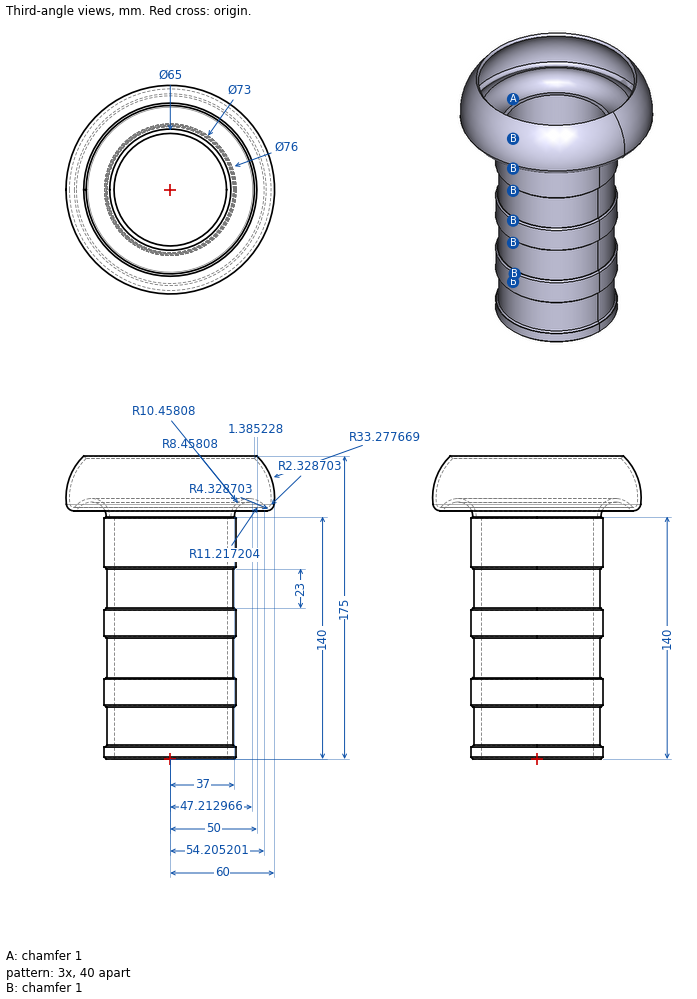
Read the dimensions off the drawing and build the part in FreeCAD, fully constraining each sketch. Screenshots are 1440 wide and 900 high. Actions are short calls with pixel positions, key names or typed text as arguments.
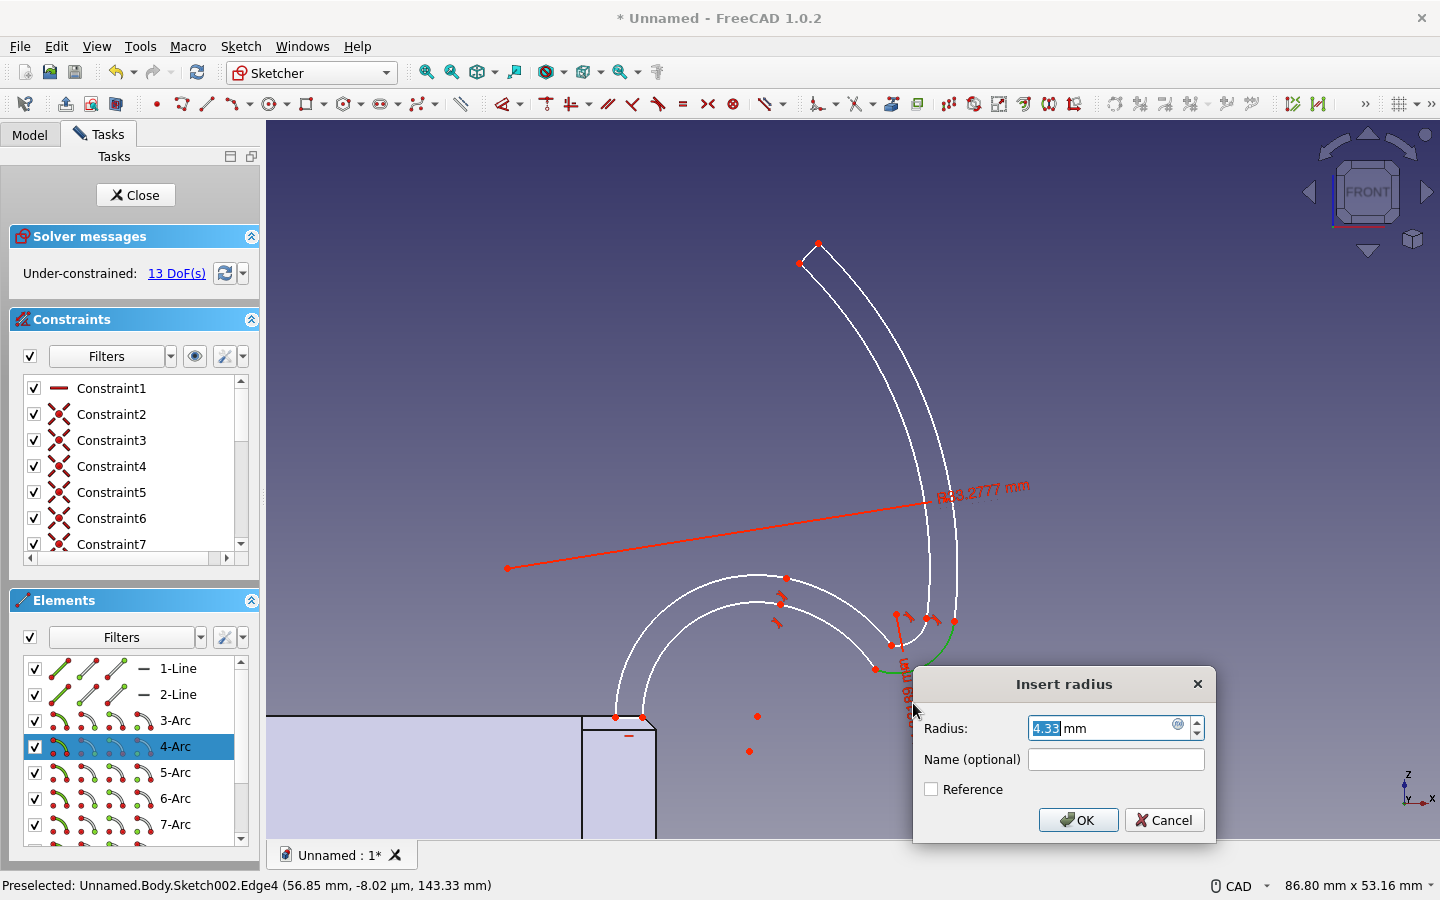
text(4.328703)
key(Return)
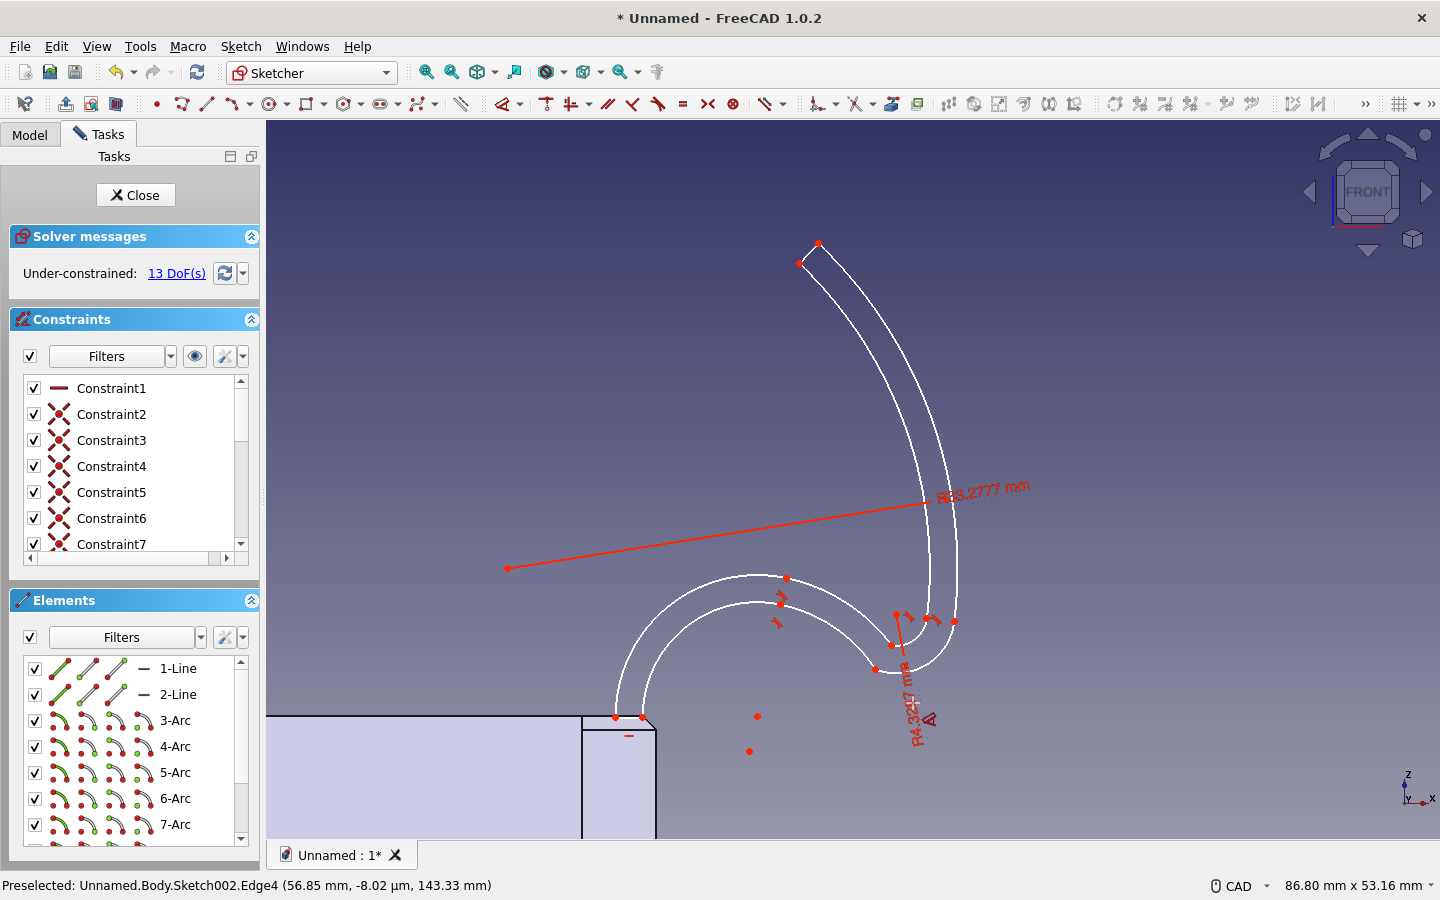
click(853, 643)
click(928, 786)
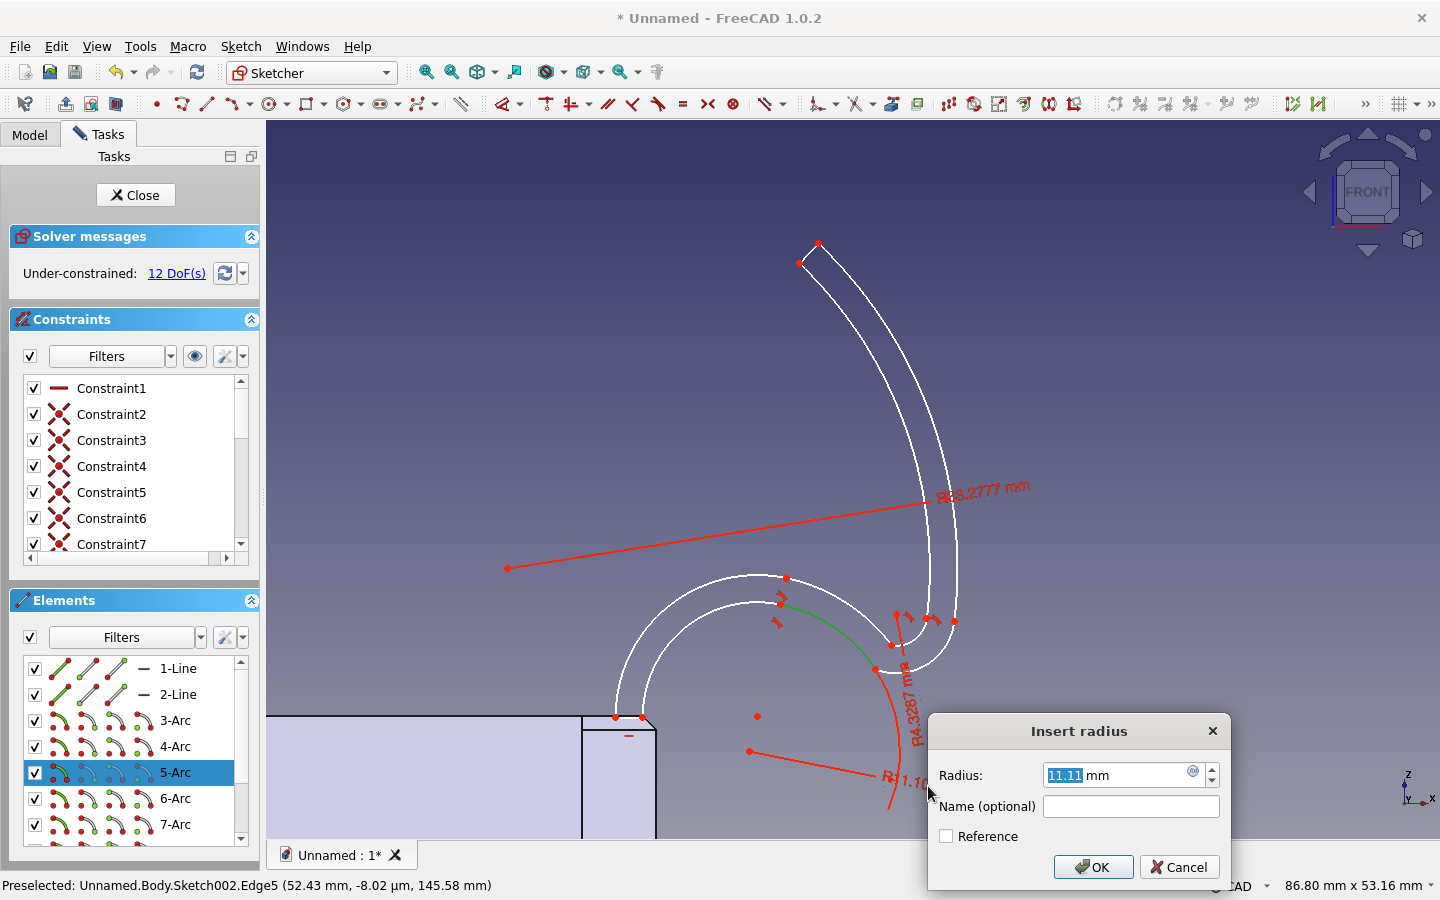
text(11.217204)
key(Return)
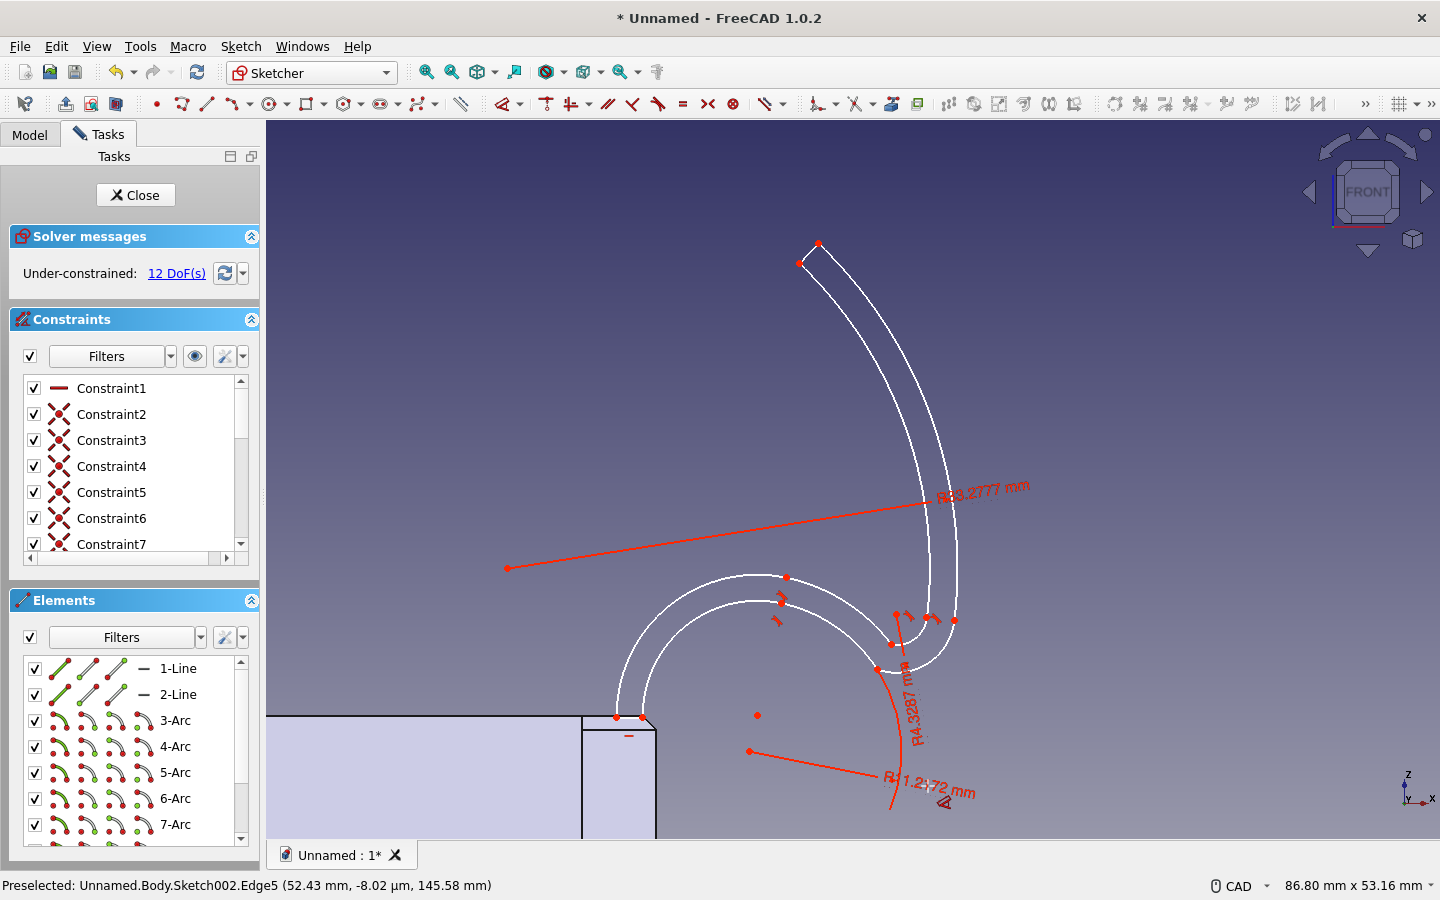
click(720, 607)
click(619, 763)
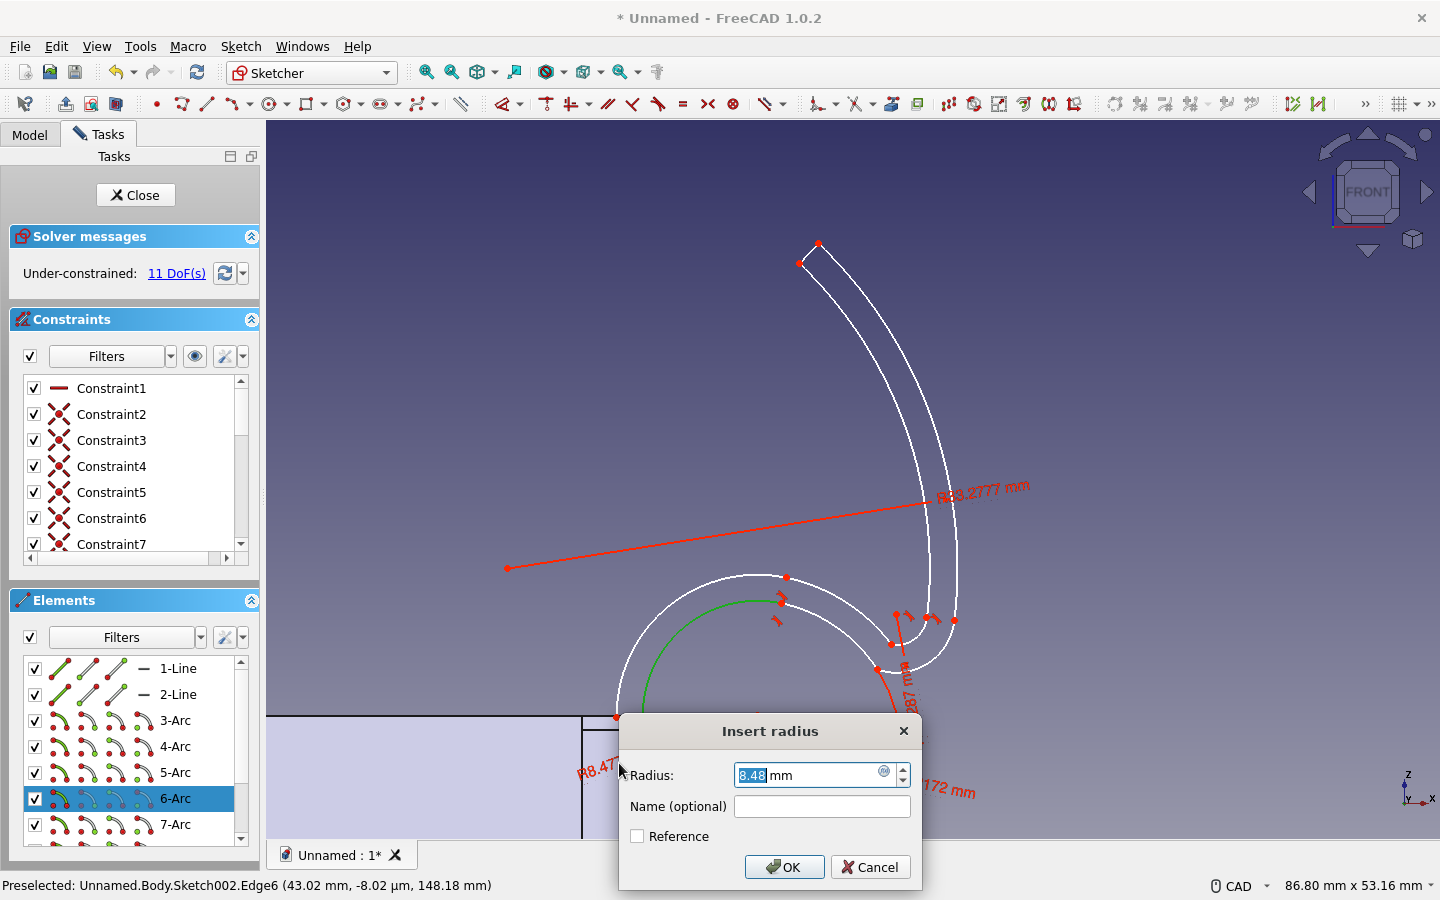
text(8.45808)
key(Return)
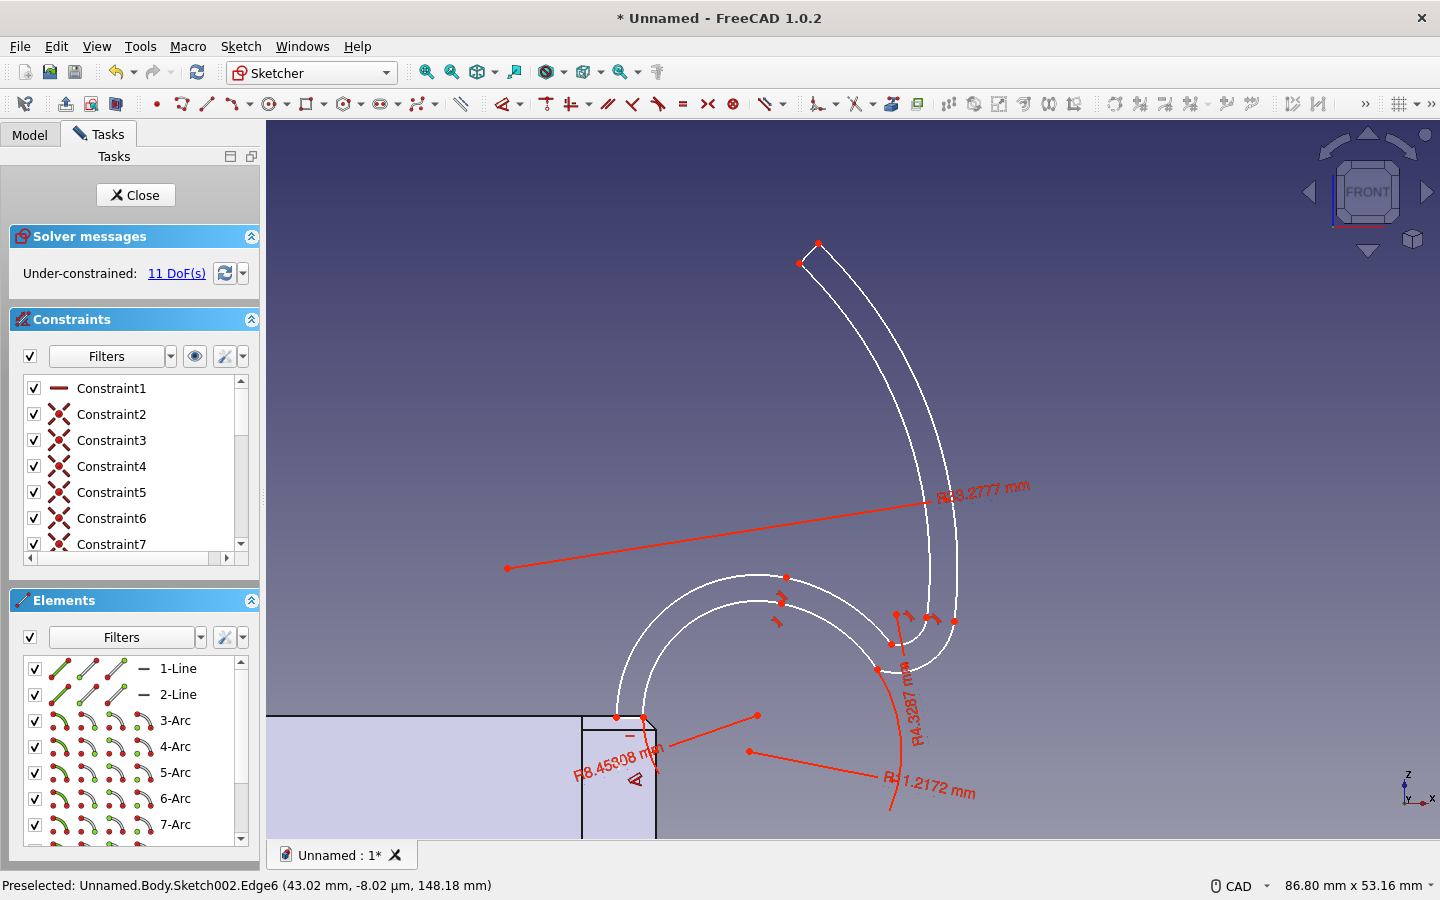
click(712, 583)
click(702, 553)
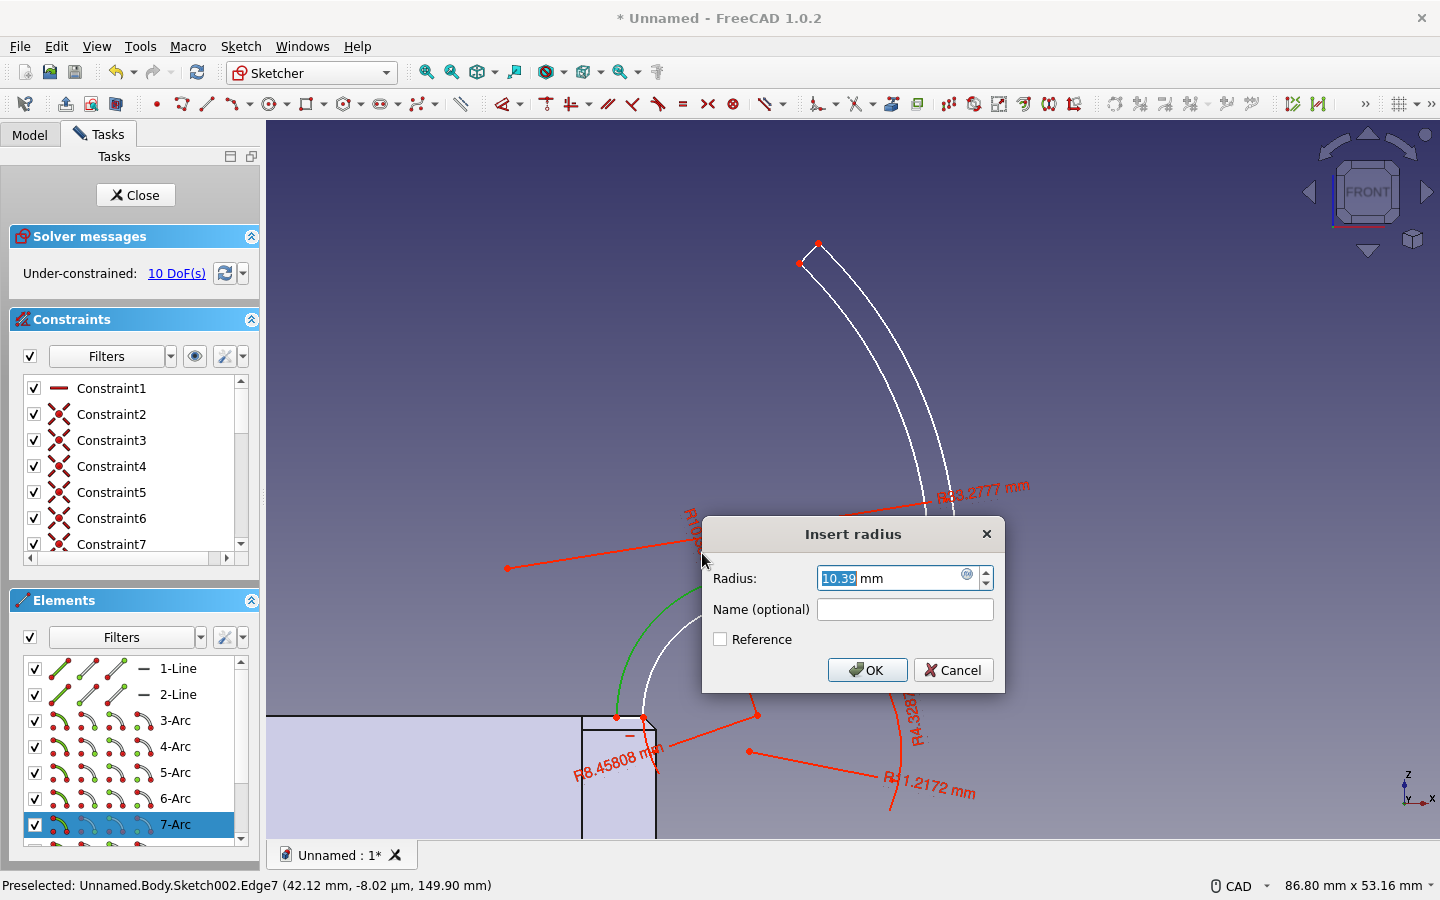
text(10.45808)
key(Return)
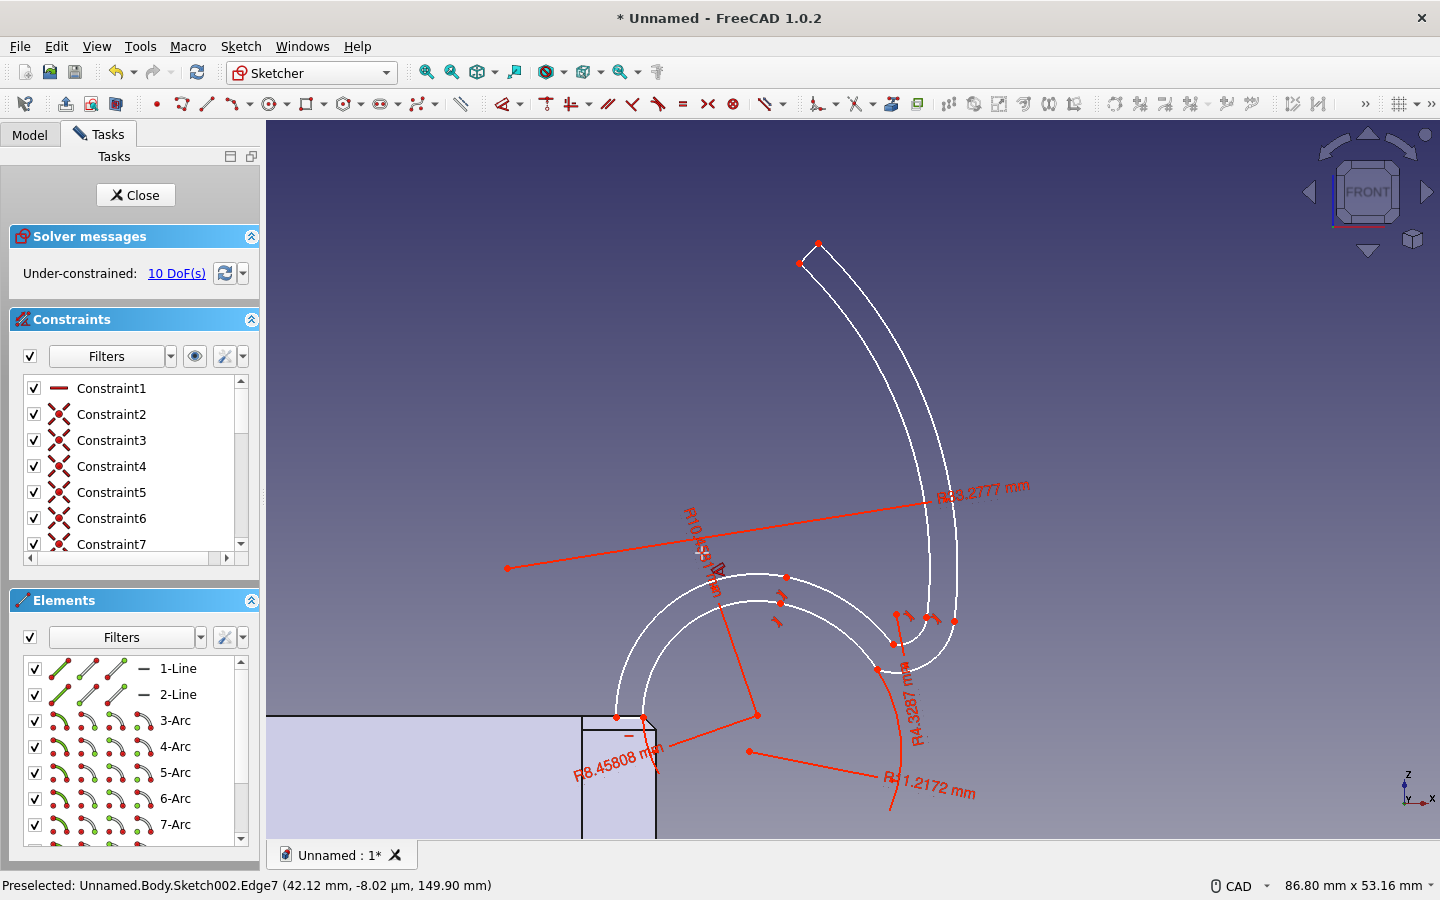
scroll(907, 643, up, 2)